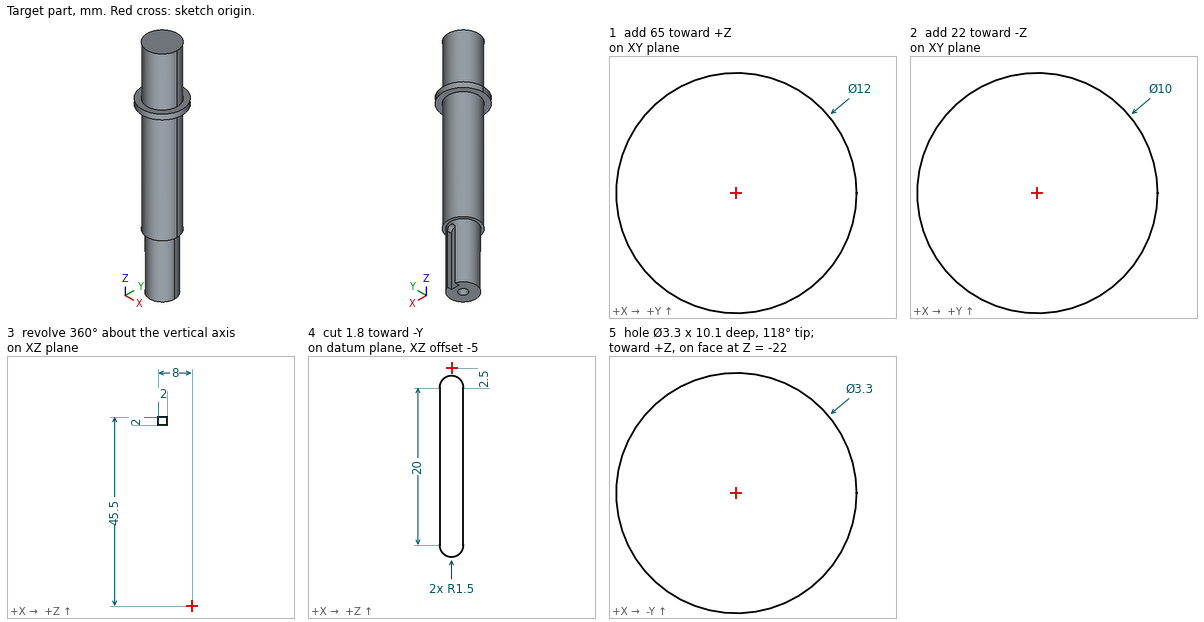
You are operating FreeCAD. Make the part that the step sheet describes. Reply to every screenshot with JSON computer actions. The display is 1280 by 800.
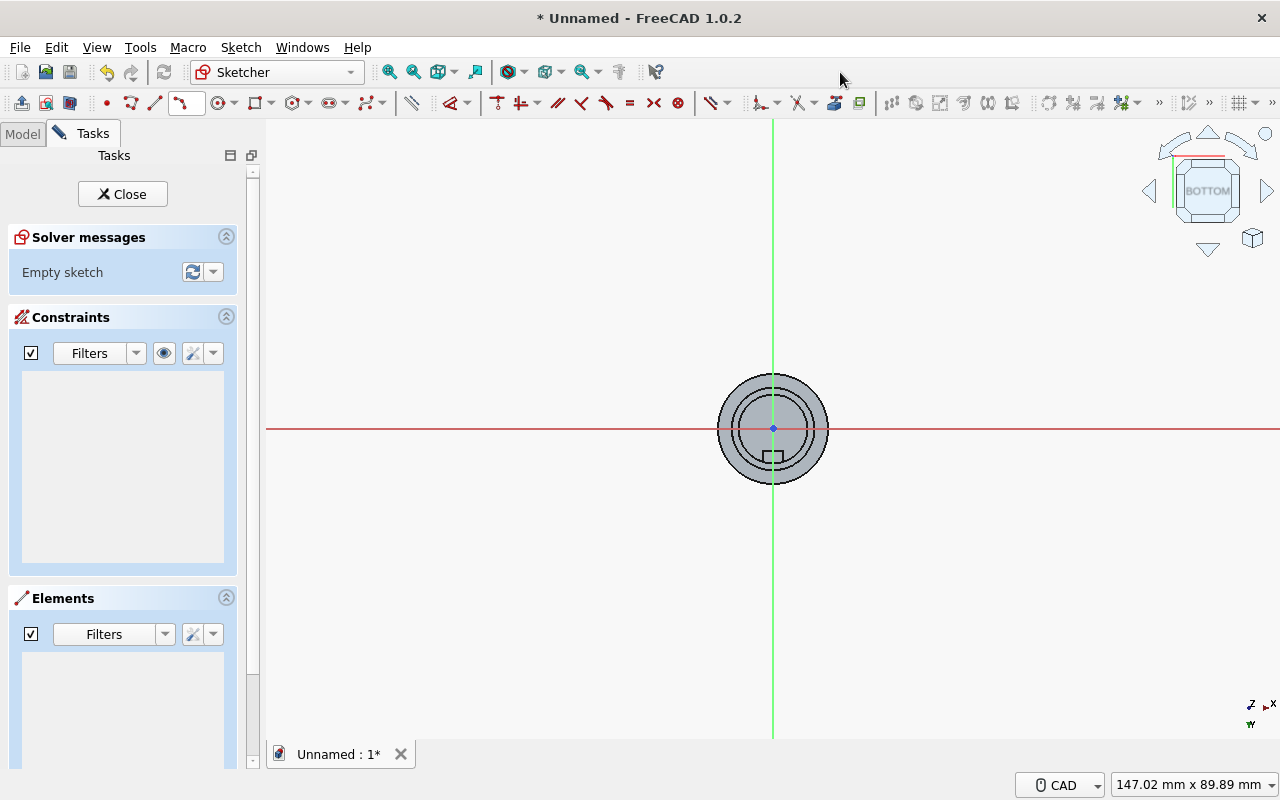
{"action": "scroll", "coordinate": [777, 429], "scroll_direction": "up", "scroll_amount": 14}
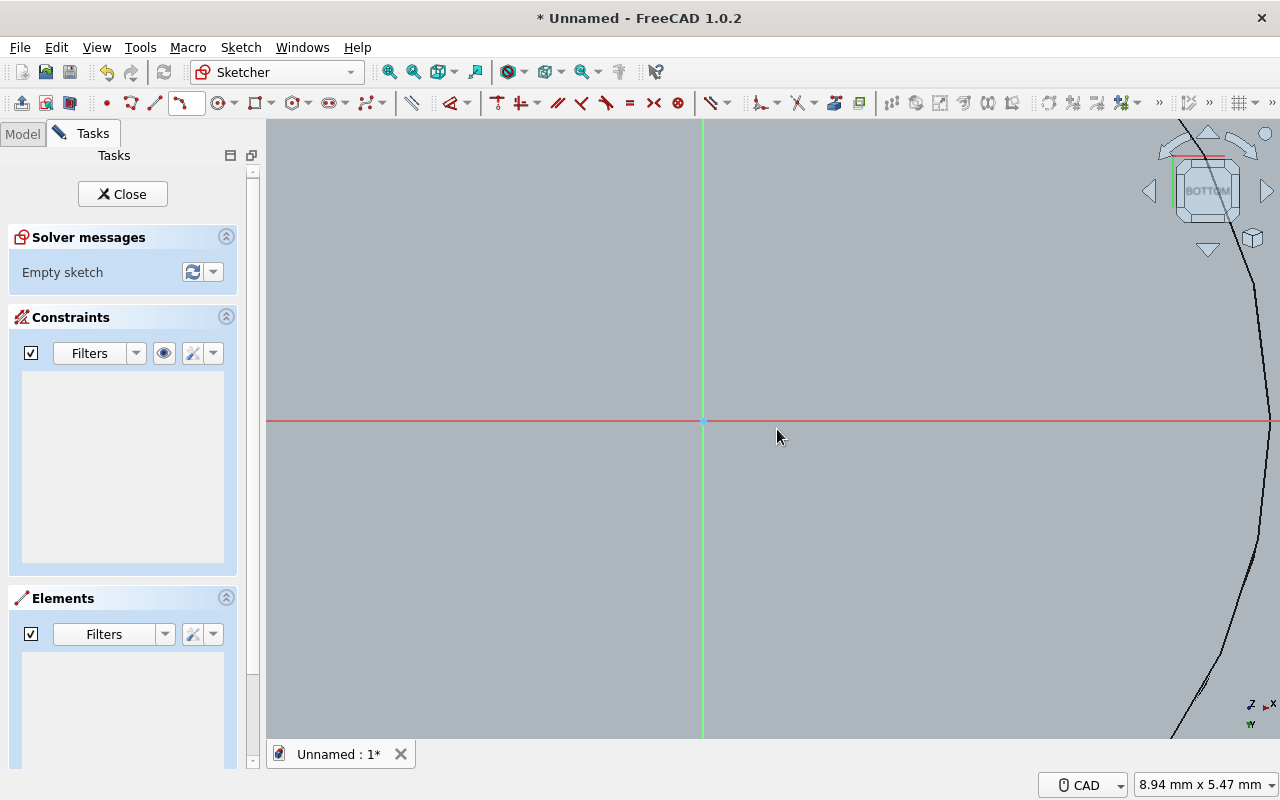
{"action": "left_click", "coordinate": [218, 104]}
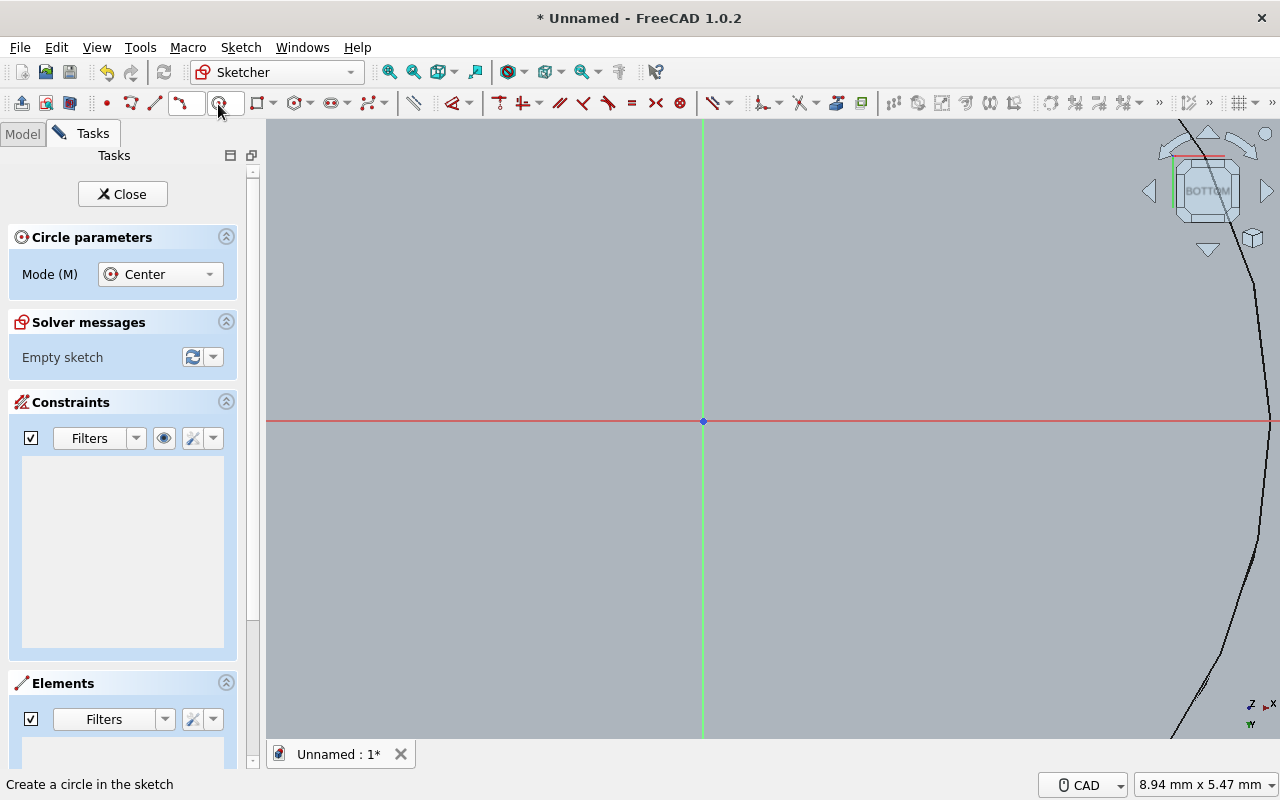
{"action": "left_click", "coordinate": [703, 421]}
{"action": "mouse_move", "coordinate": [836, 289]}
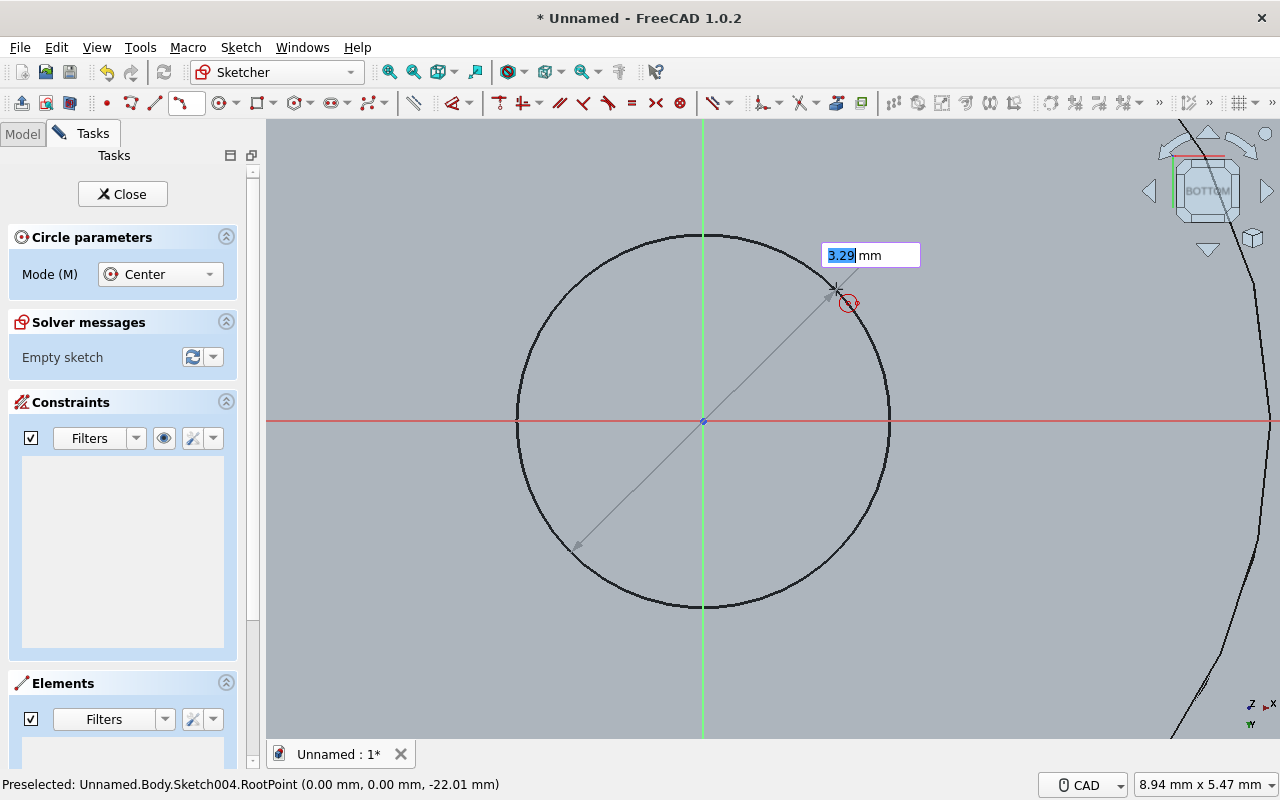
{"action": "type", "text": "3.3"}
{"action": "key", "text": "Return"}
{"action": "key", "text": "Escape"}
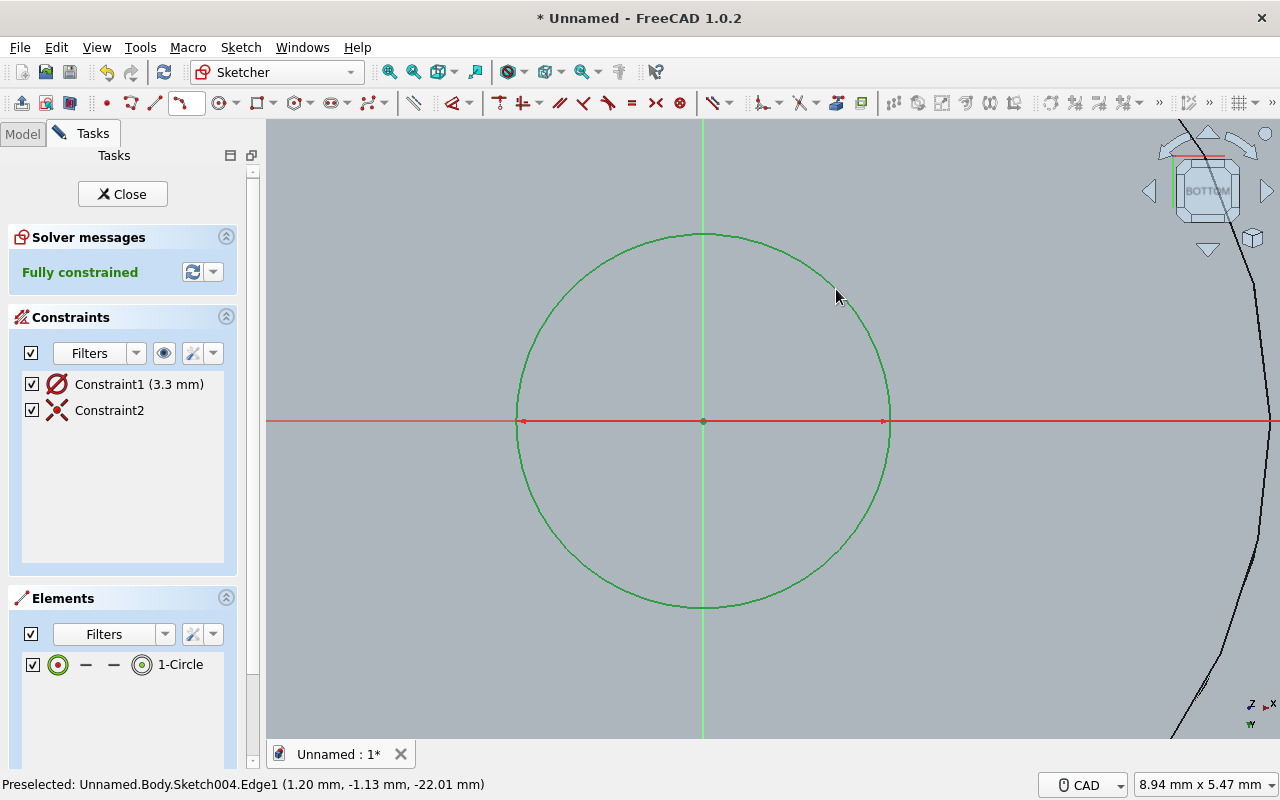
{"action": "left_click", "coordinate": [123, 194]}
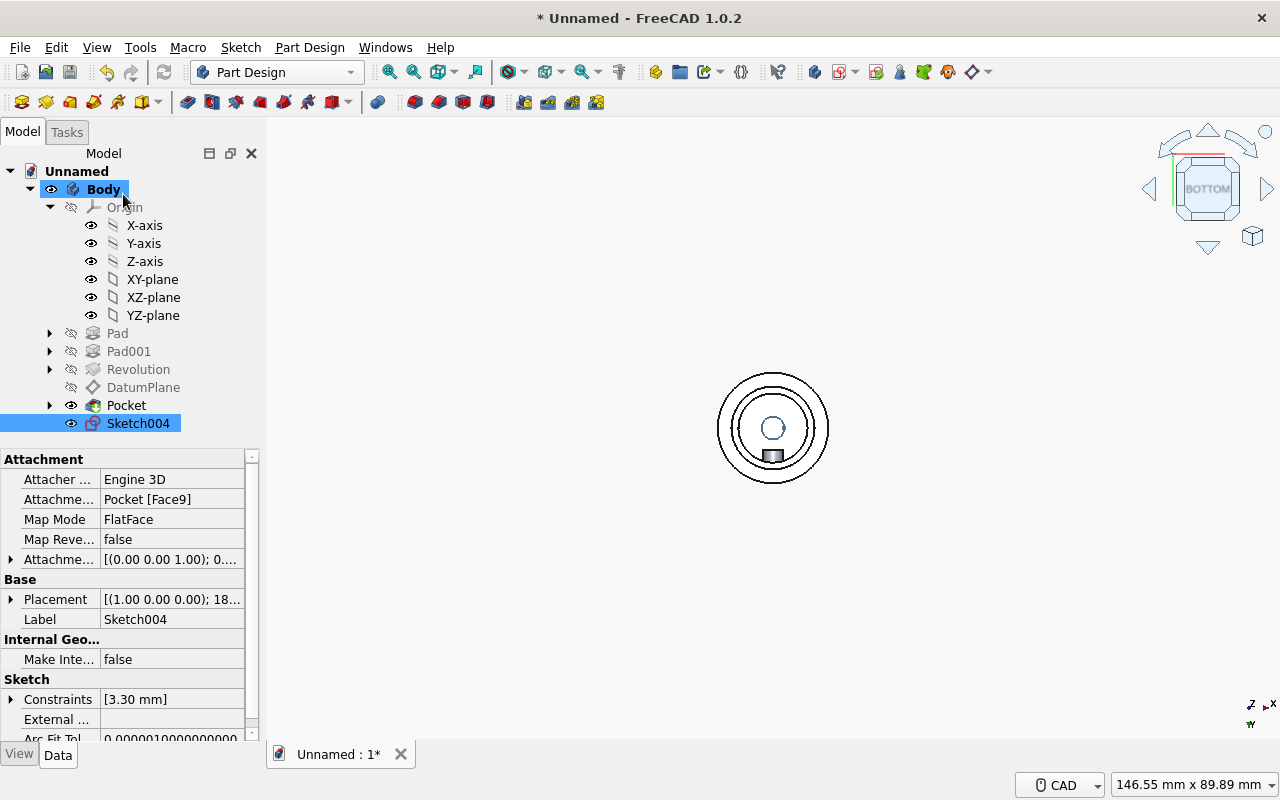
{"action": "left_click", "coordinate": [212, 102]}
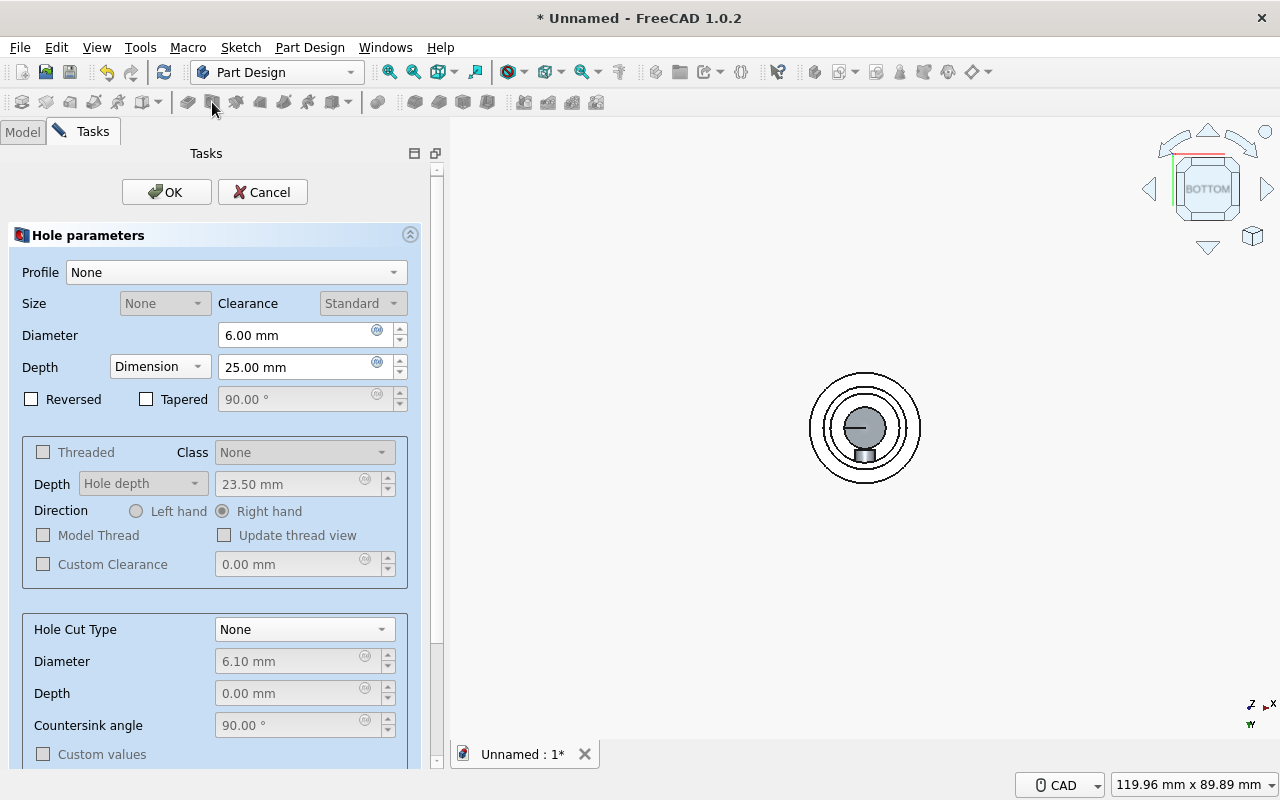
{"action": "triple_click", "coordinate": [305, 335]}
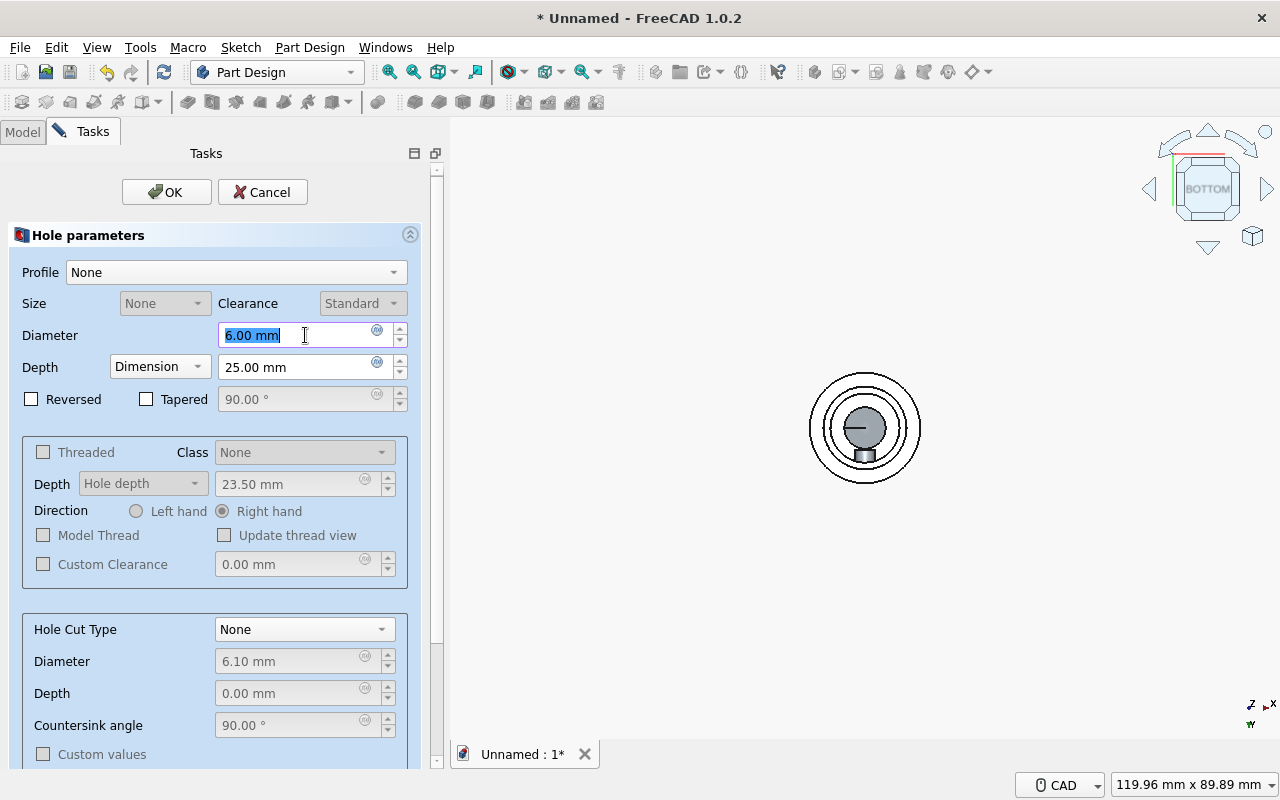
{"action": "type", "text": "3.3"}
{"action": "key", "text": "Tab"}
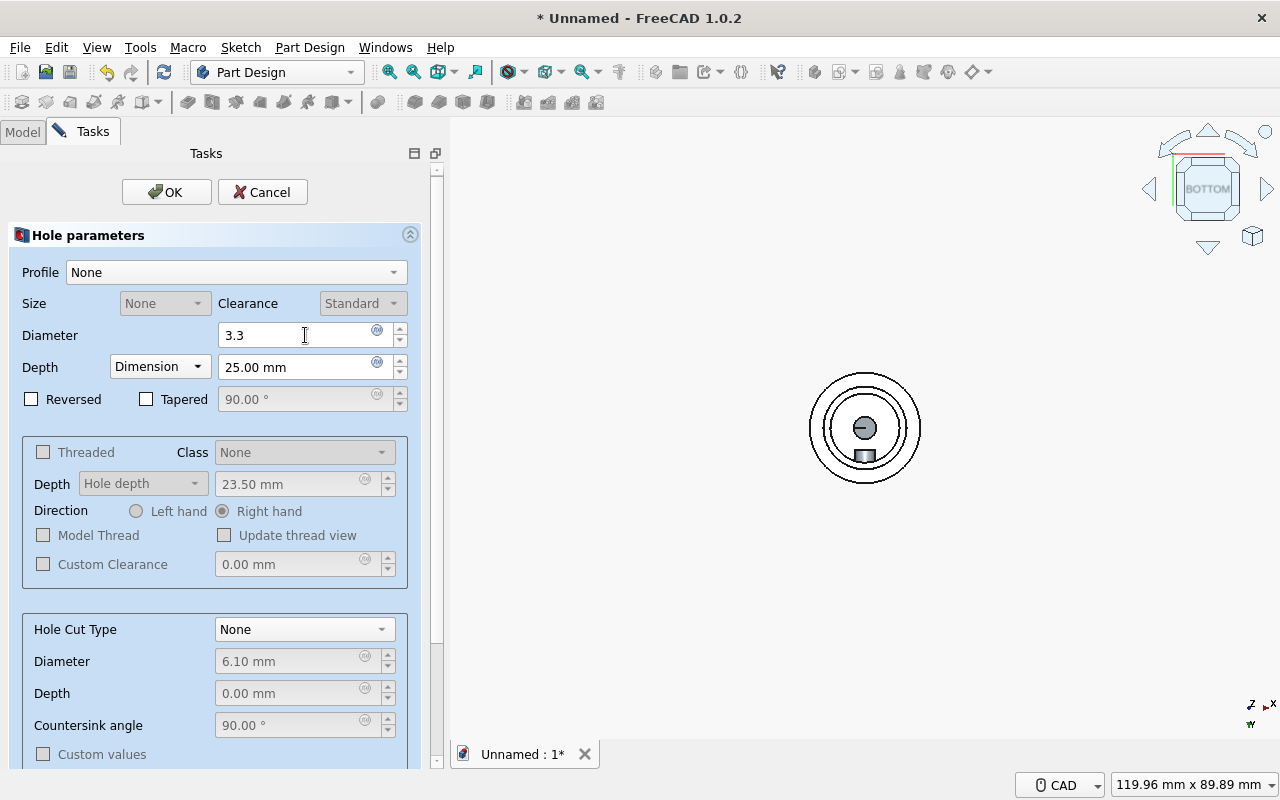
{"action": "triple_click", "coordinate": [305, 367]}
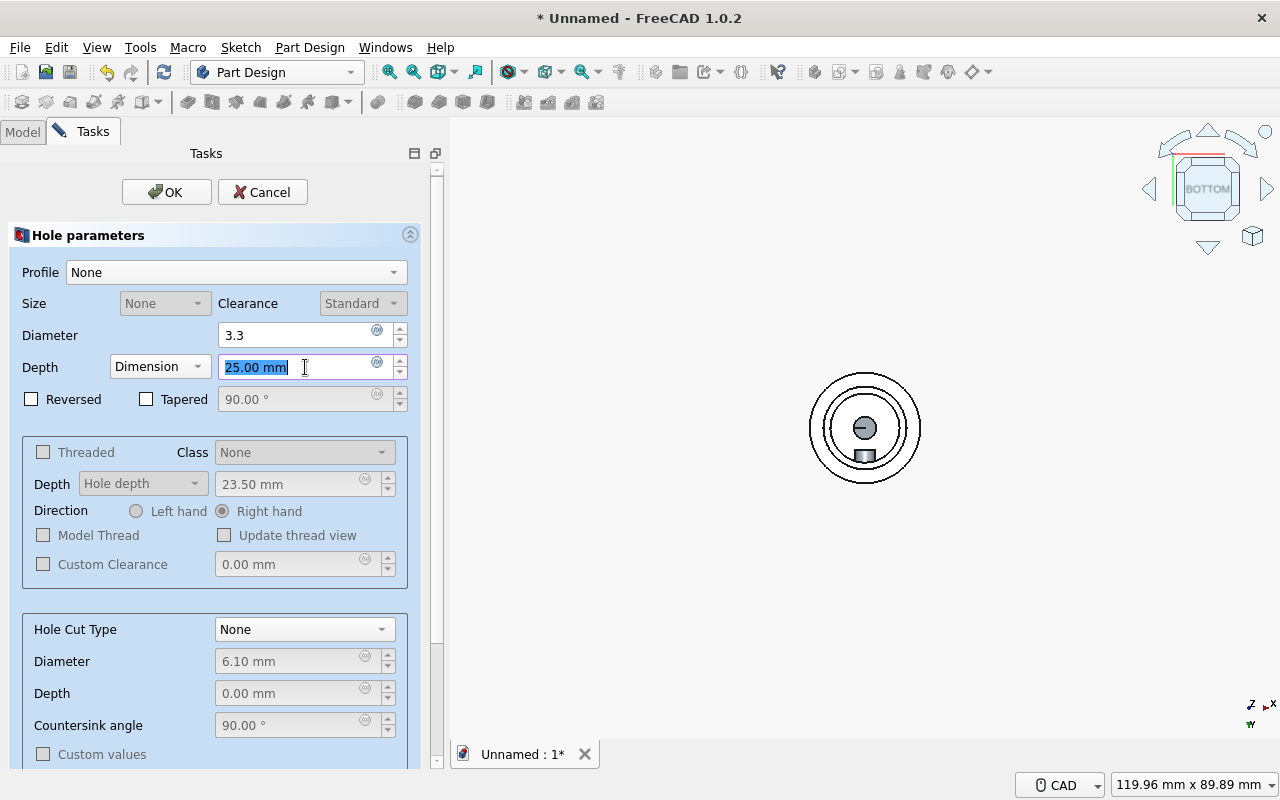
{"action": "type", "text": "10.1"}
{"action": "key", "text": "Tab"}